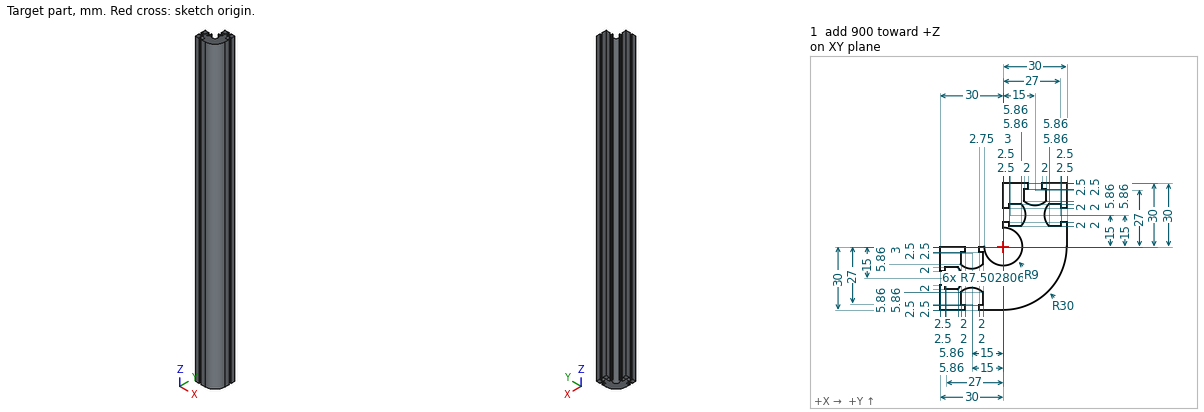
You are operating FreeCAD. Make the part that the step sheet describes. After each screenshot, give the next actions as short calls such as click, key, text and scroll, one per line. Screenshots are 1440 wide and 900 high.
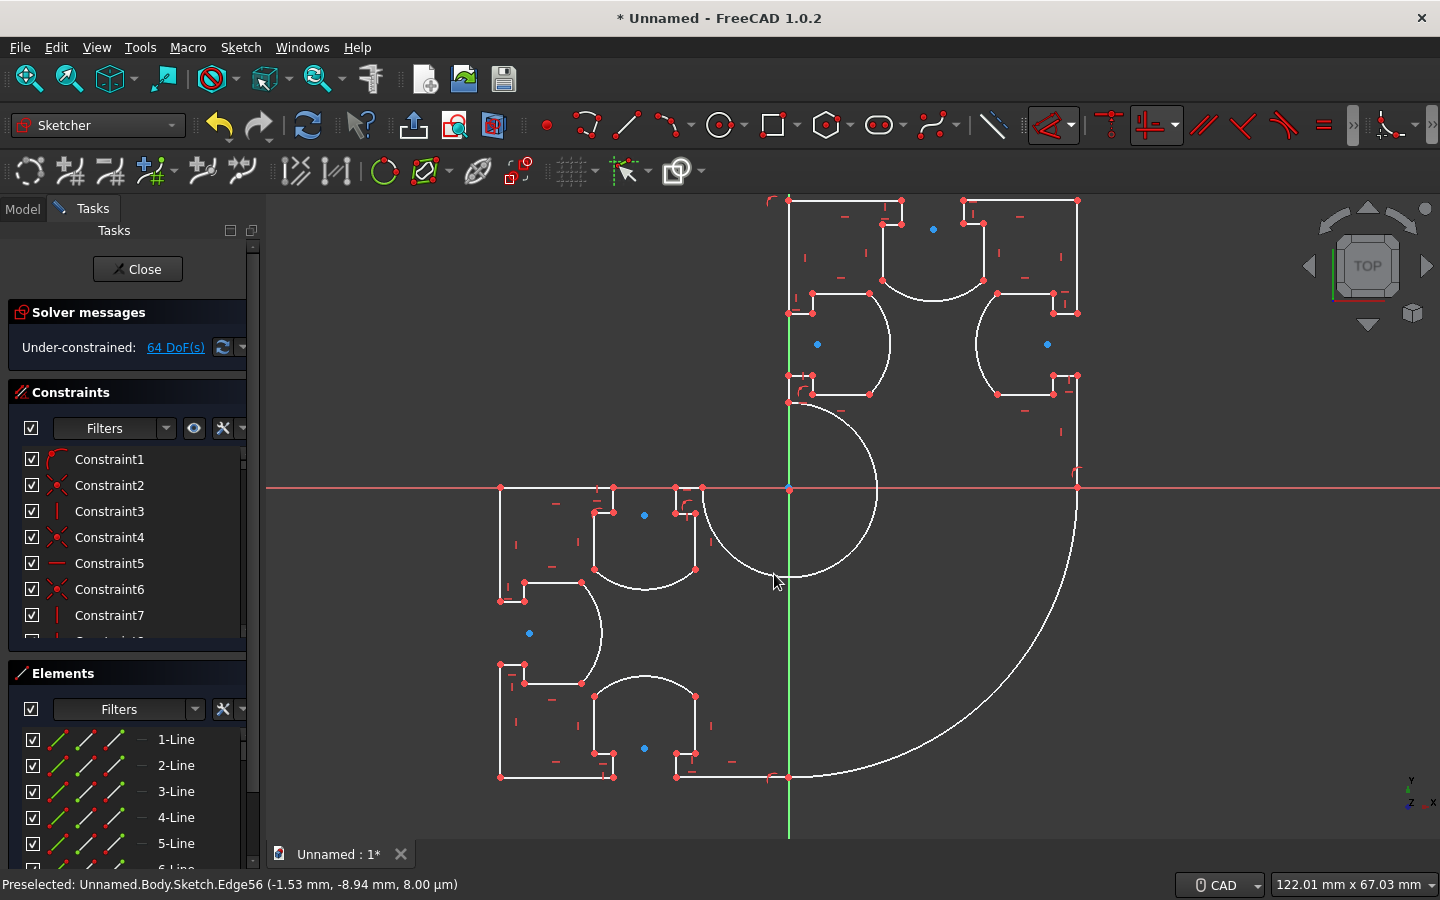
drag(779, 478, 800, 500)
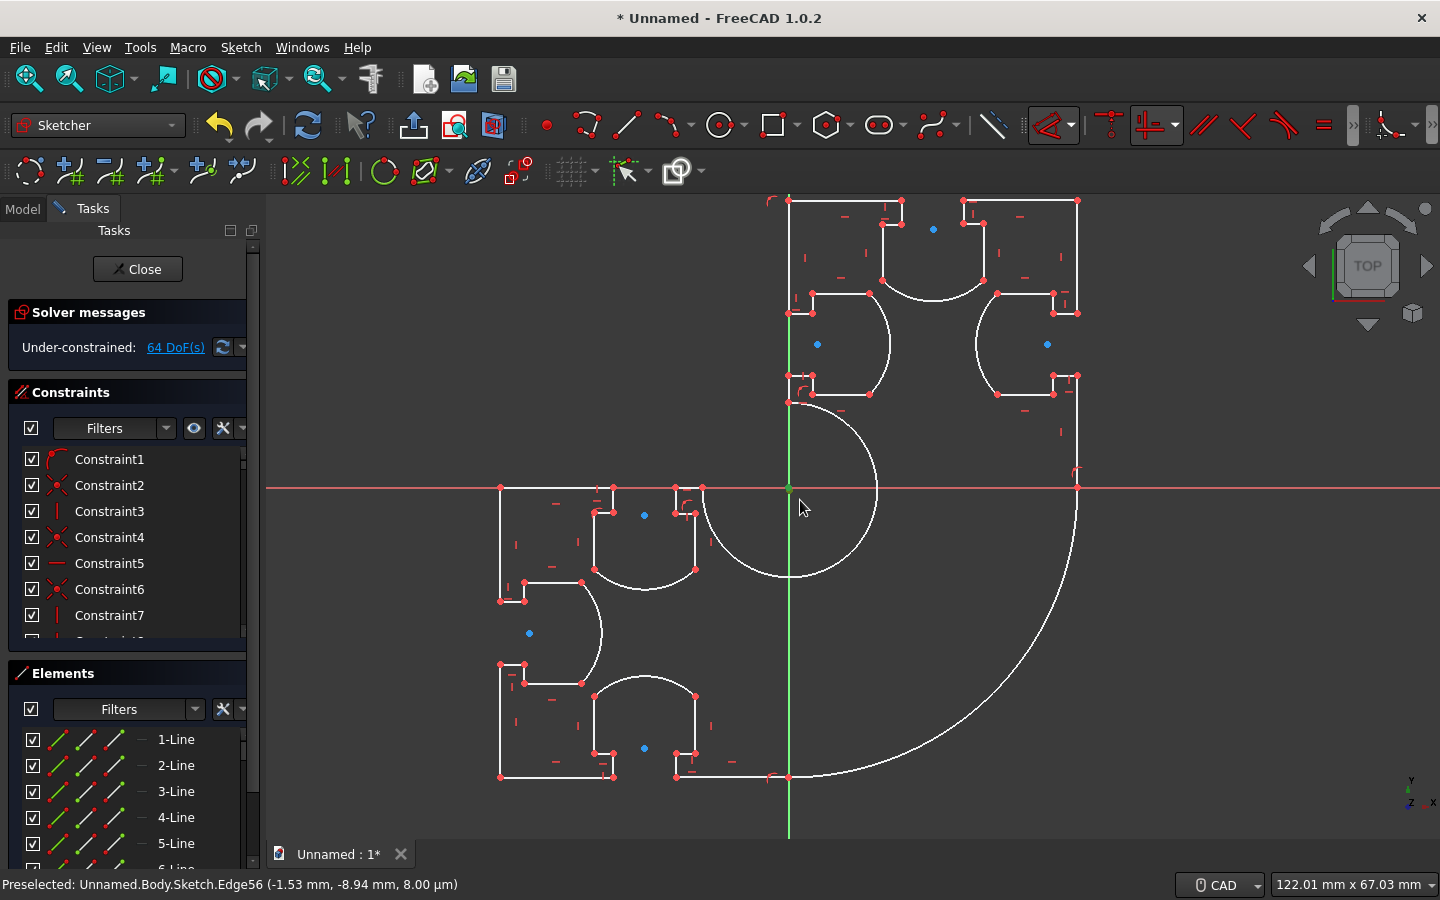
click(1110, 126)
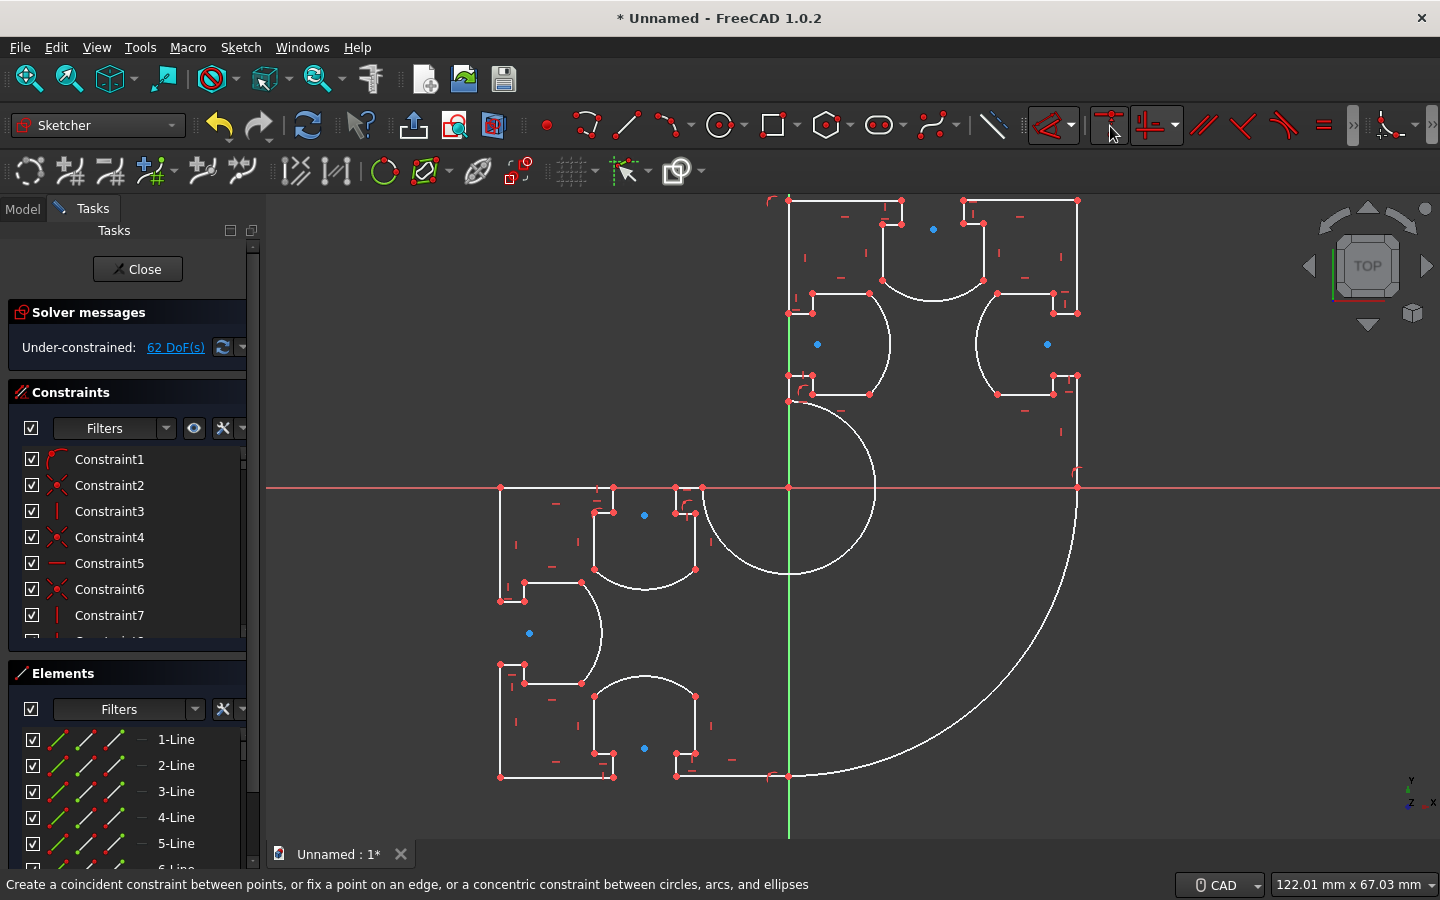
click(623, 586)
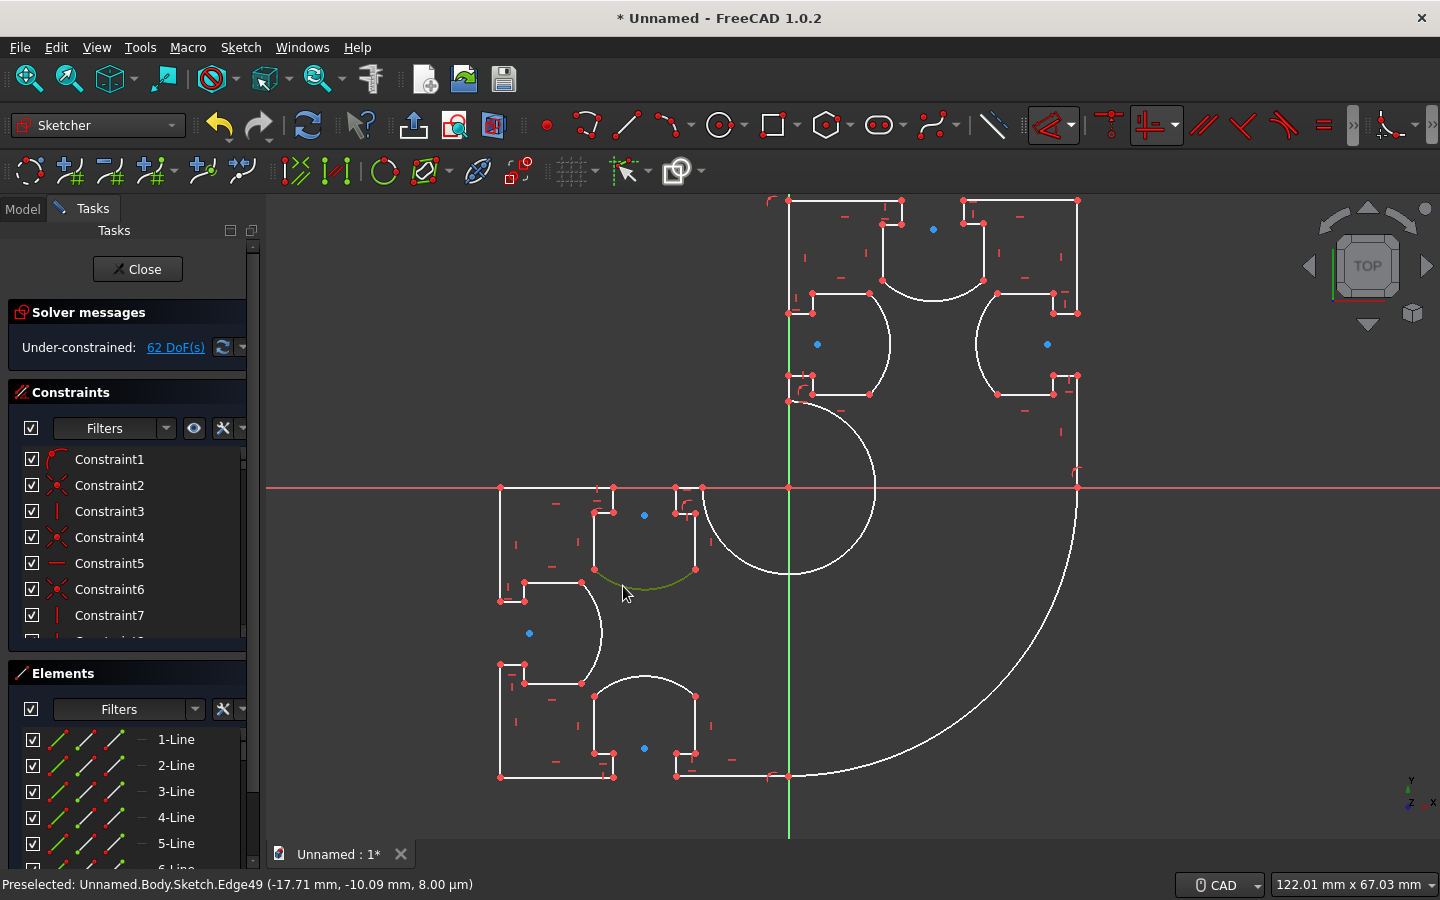
click(598, 655)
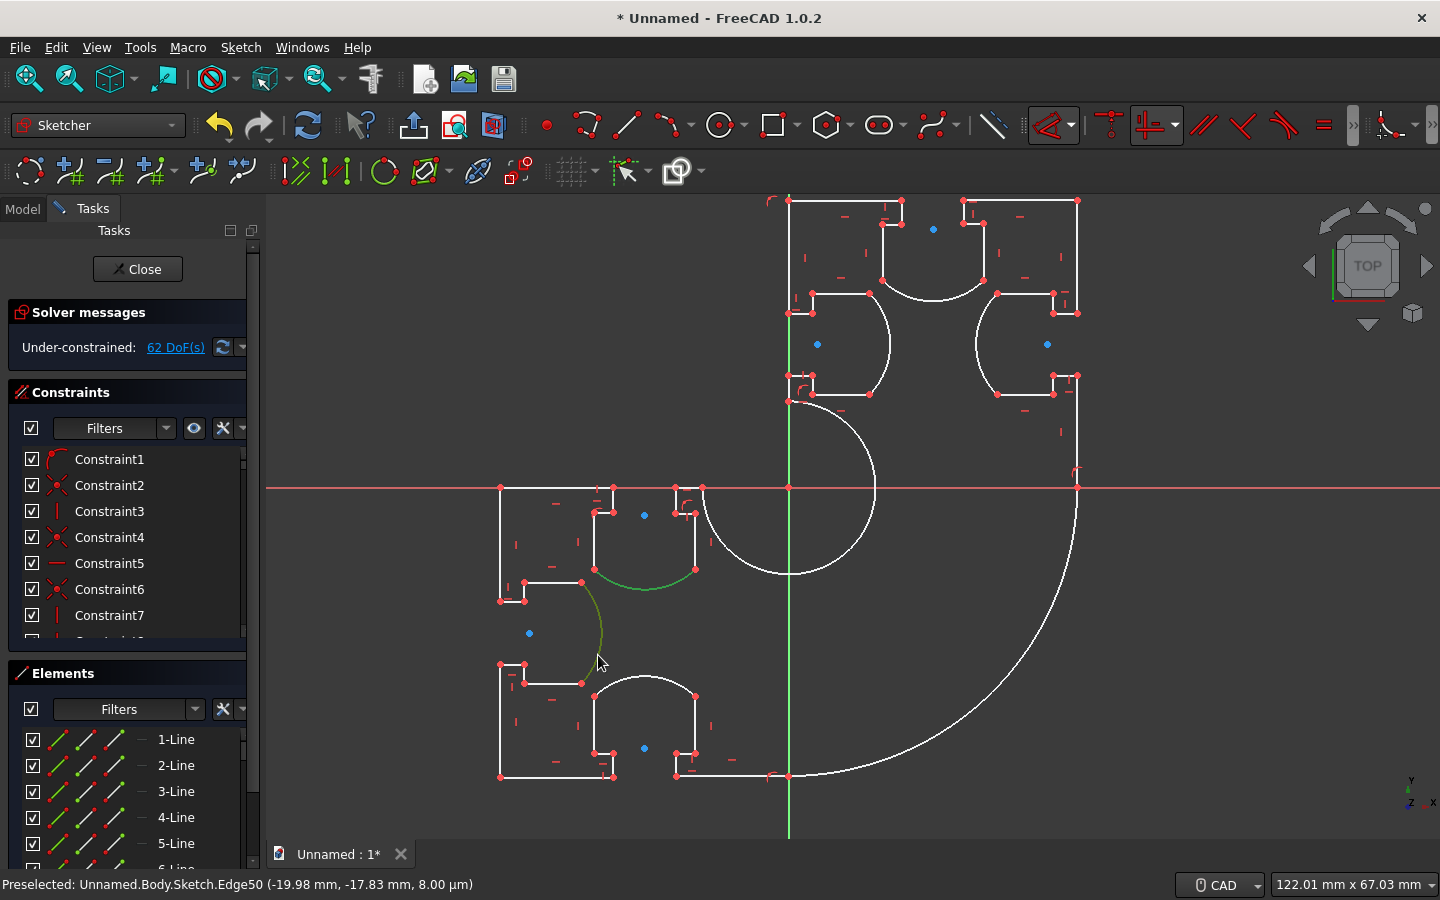
click(667, 680)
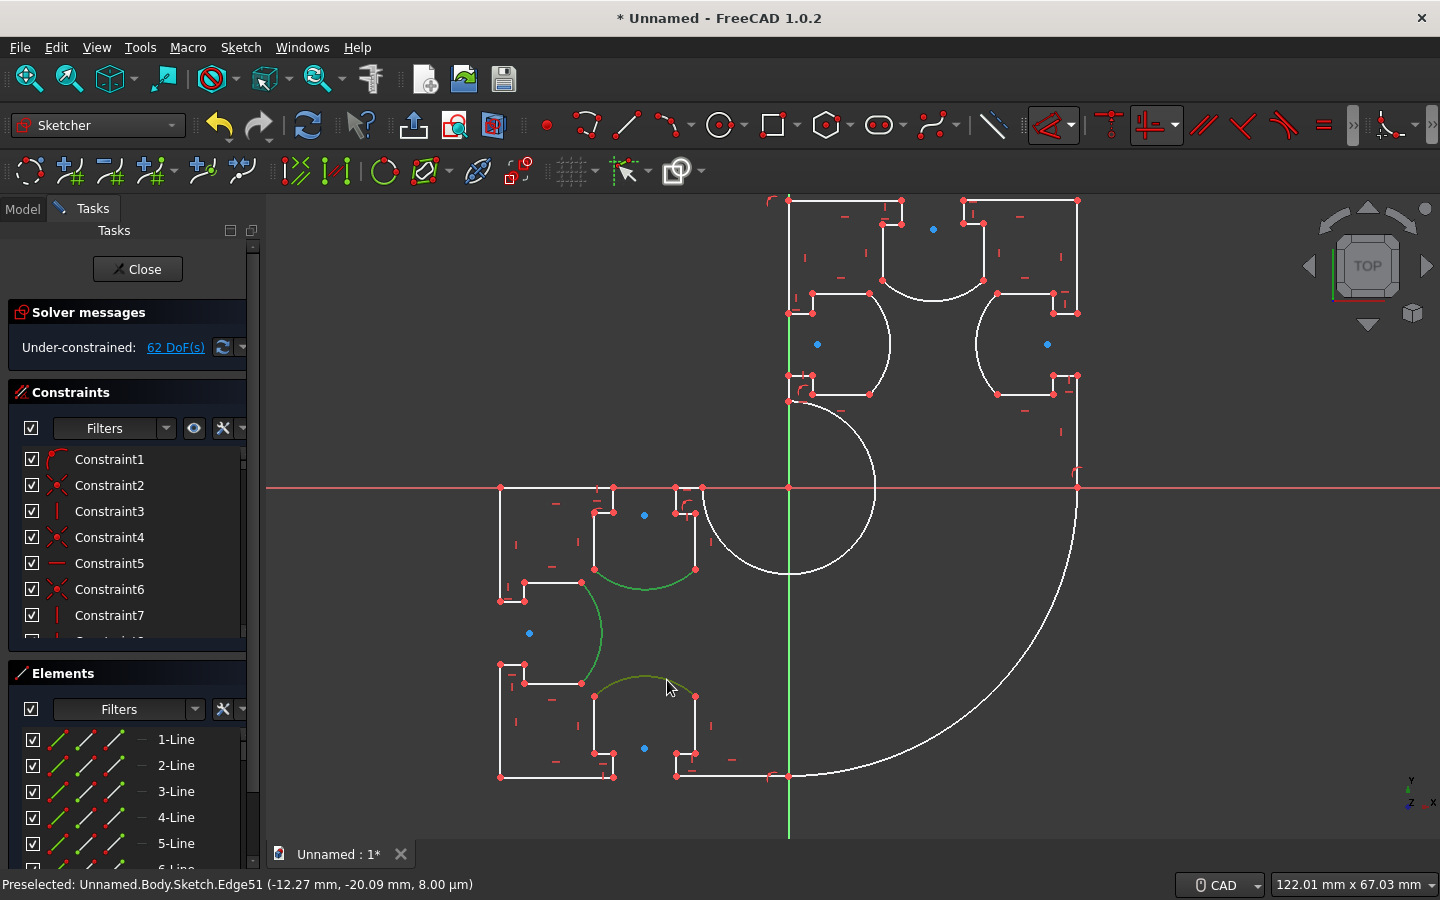
click(980, 322)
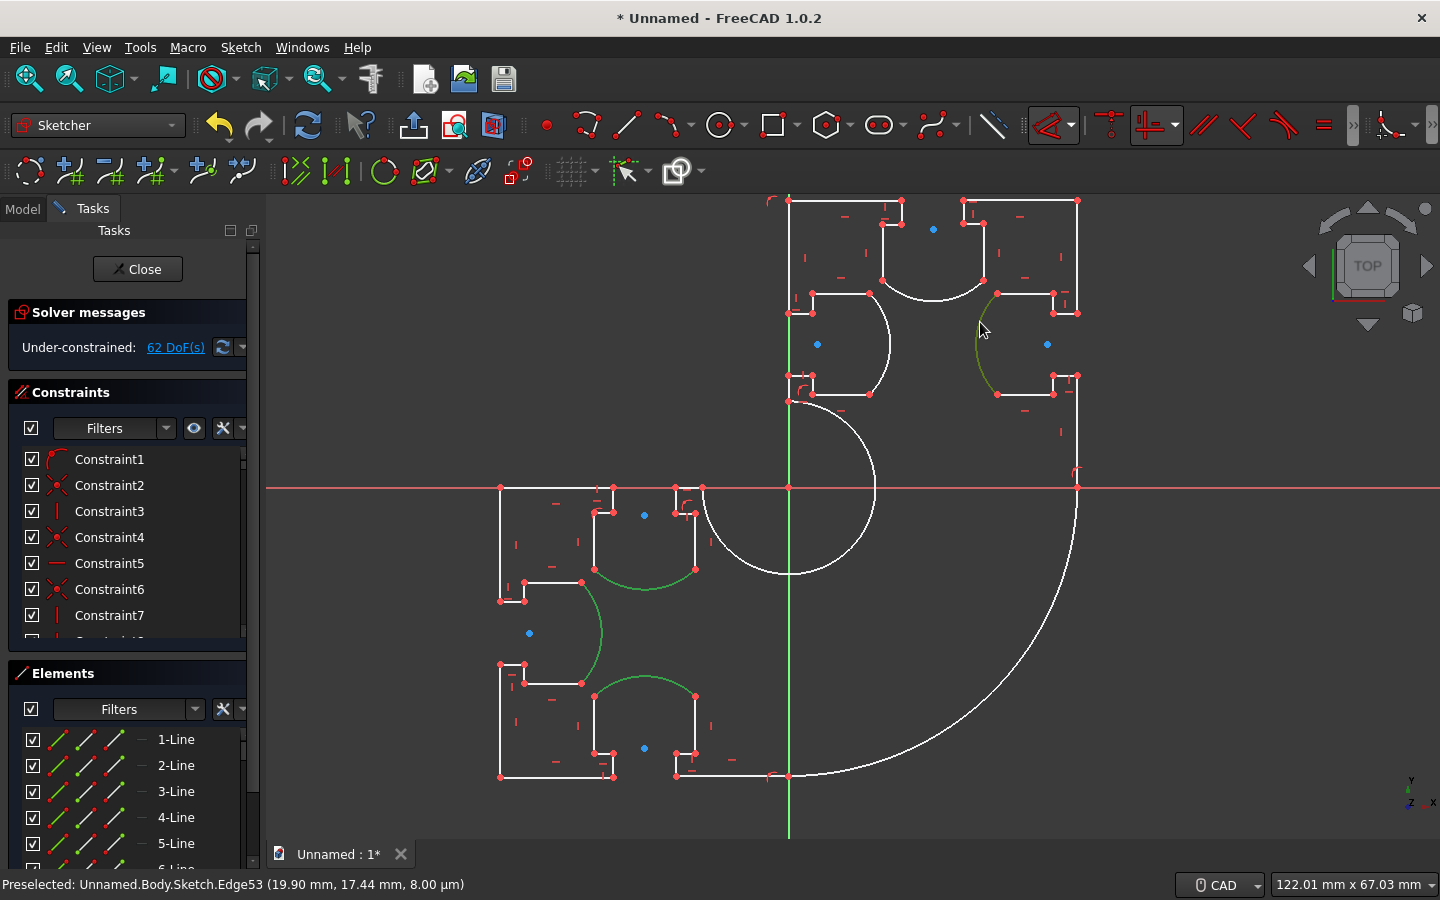
click(911, 298)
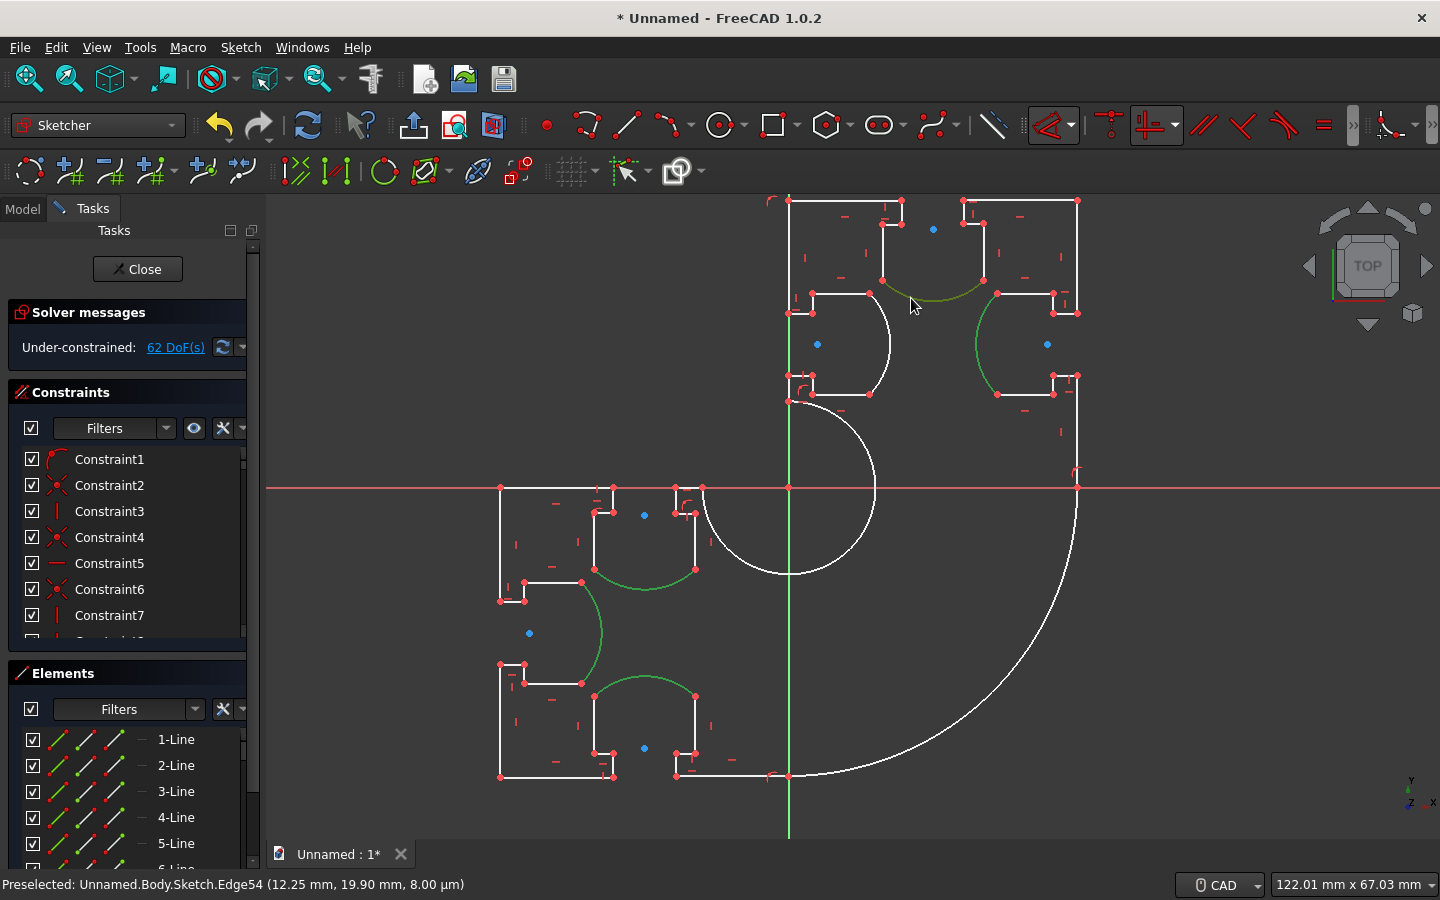
click(887, 366)